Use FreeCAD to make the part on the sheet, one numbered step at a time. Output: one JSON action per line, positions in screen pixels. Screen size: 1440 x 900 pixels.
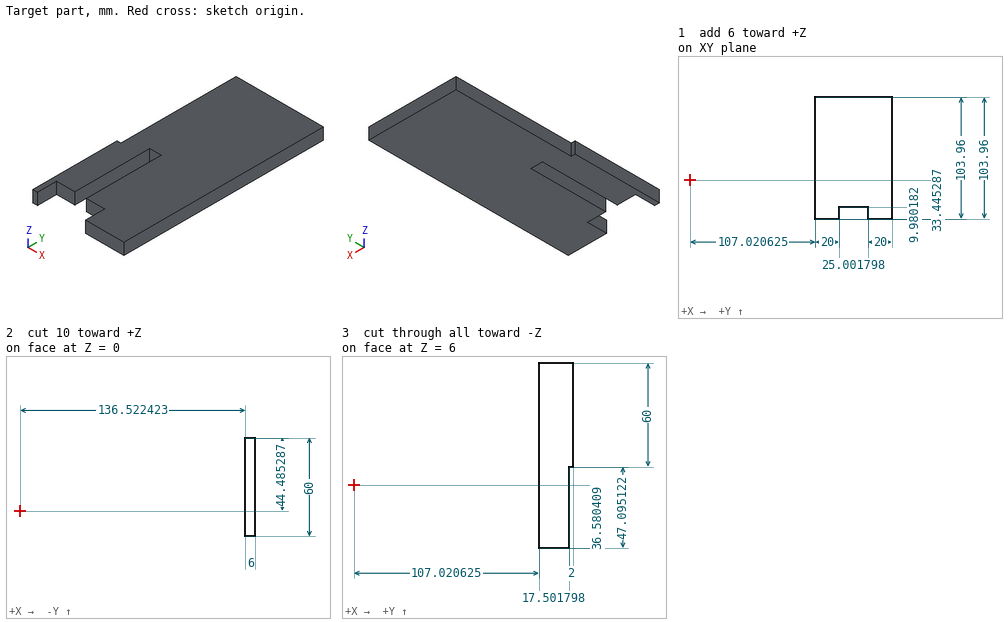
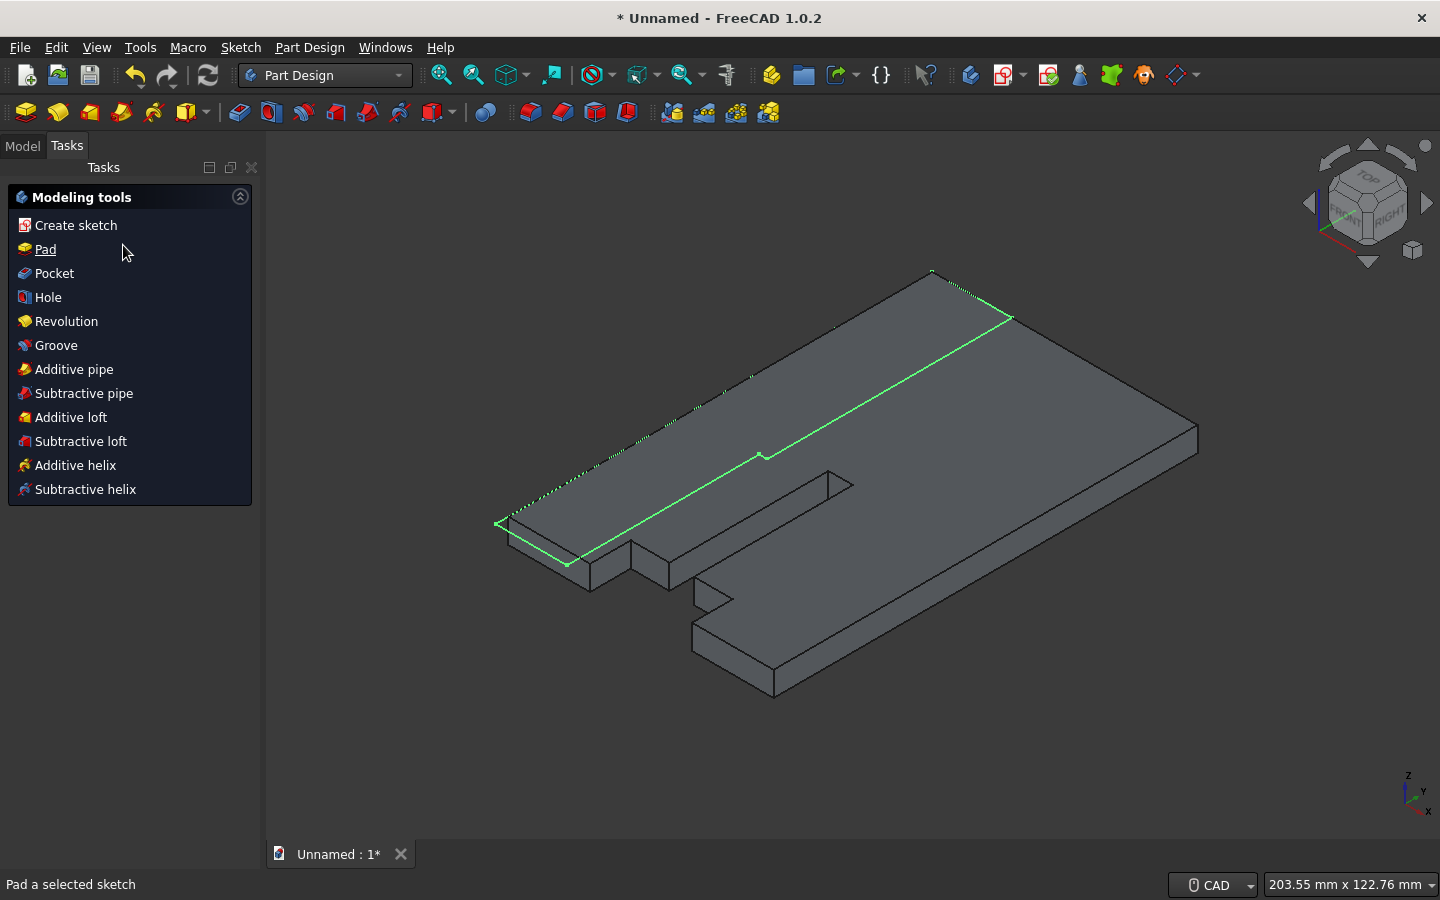
{"action": "left_click", "coordinate": [240, 112]}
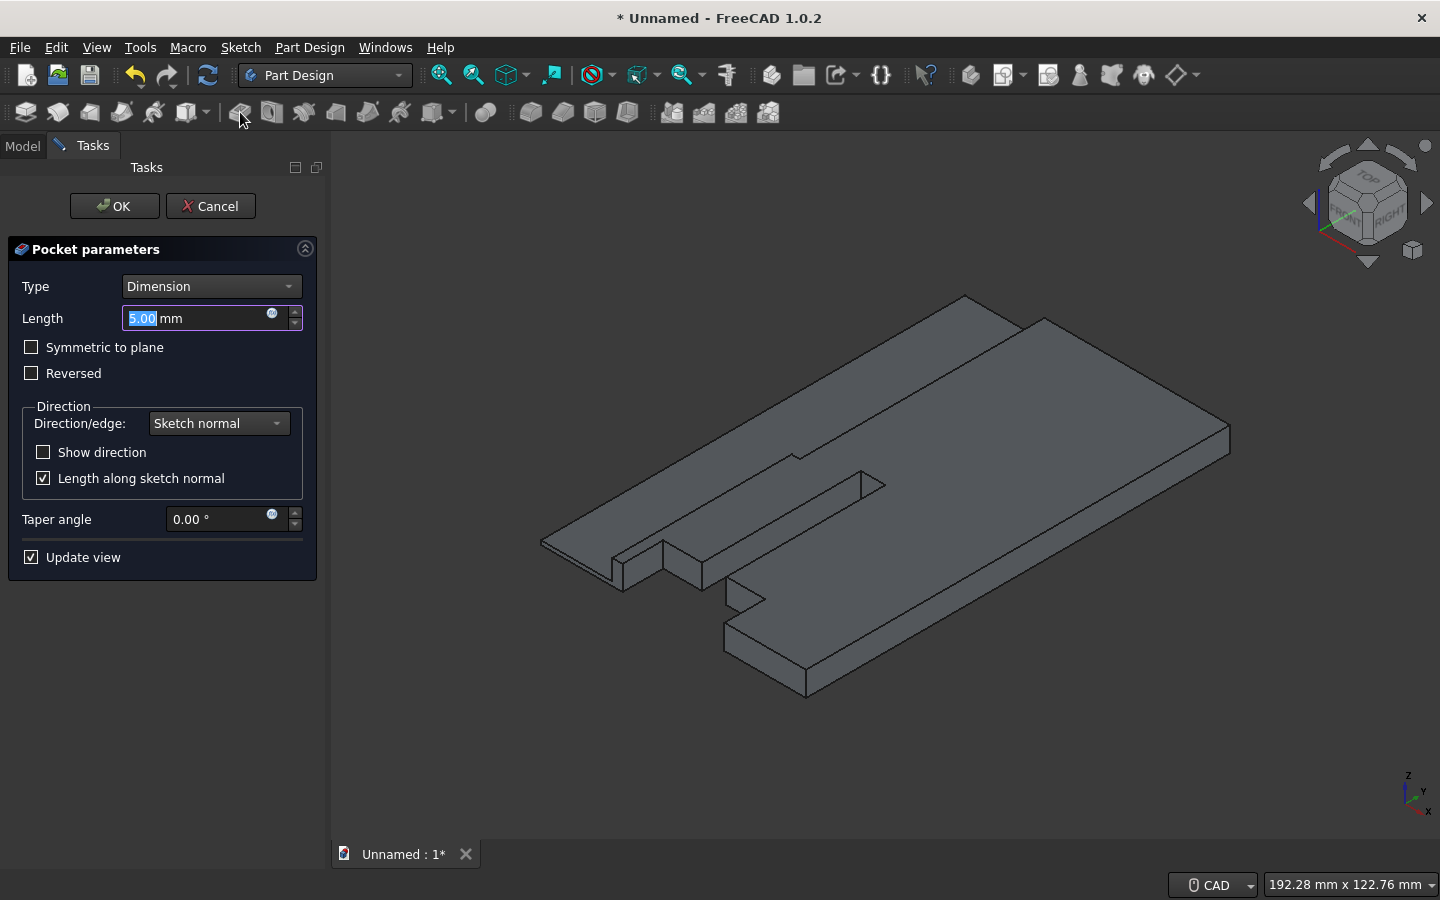
{"action": "left_click", "coordinate": [212, 286]}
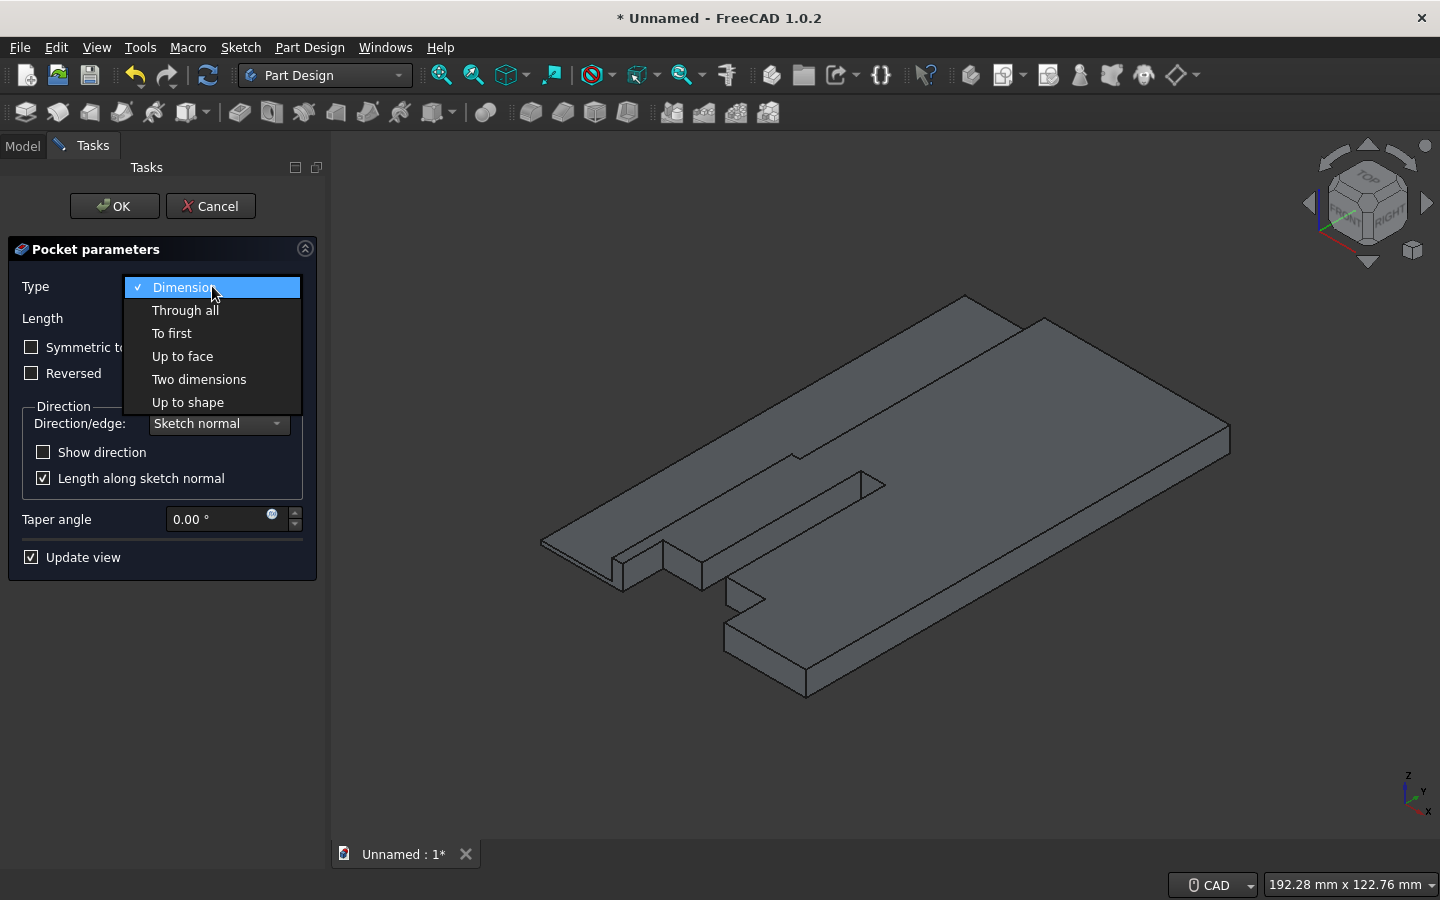
{"action": "left_click", "coordinate": [212, 310]}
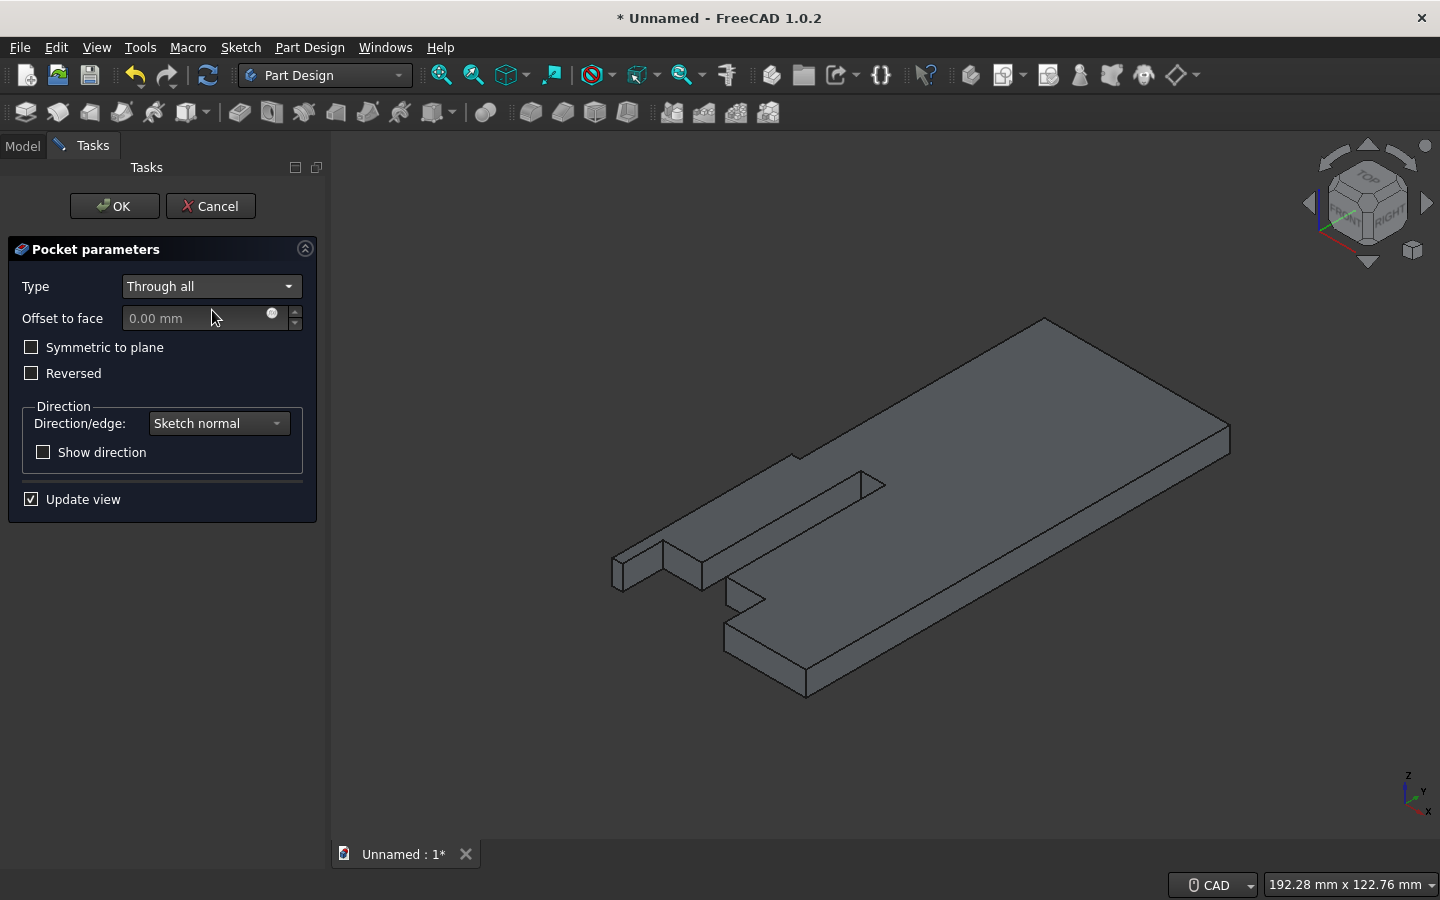
{"action": "left_click", "coordinate": [115, 206]}